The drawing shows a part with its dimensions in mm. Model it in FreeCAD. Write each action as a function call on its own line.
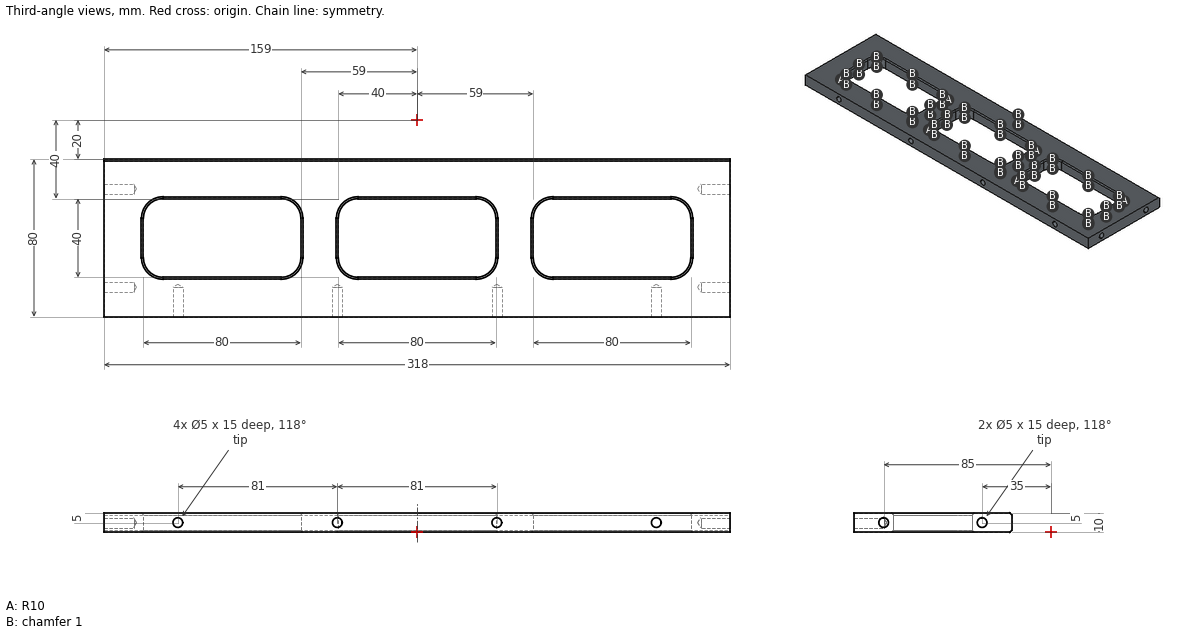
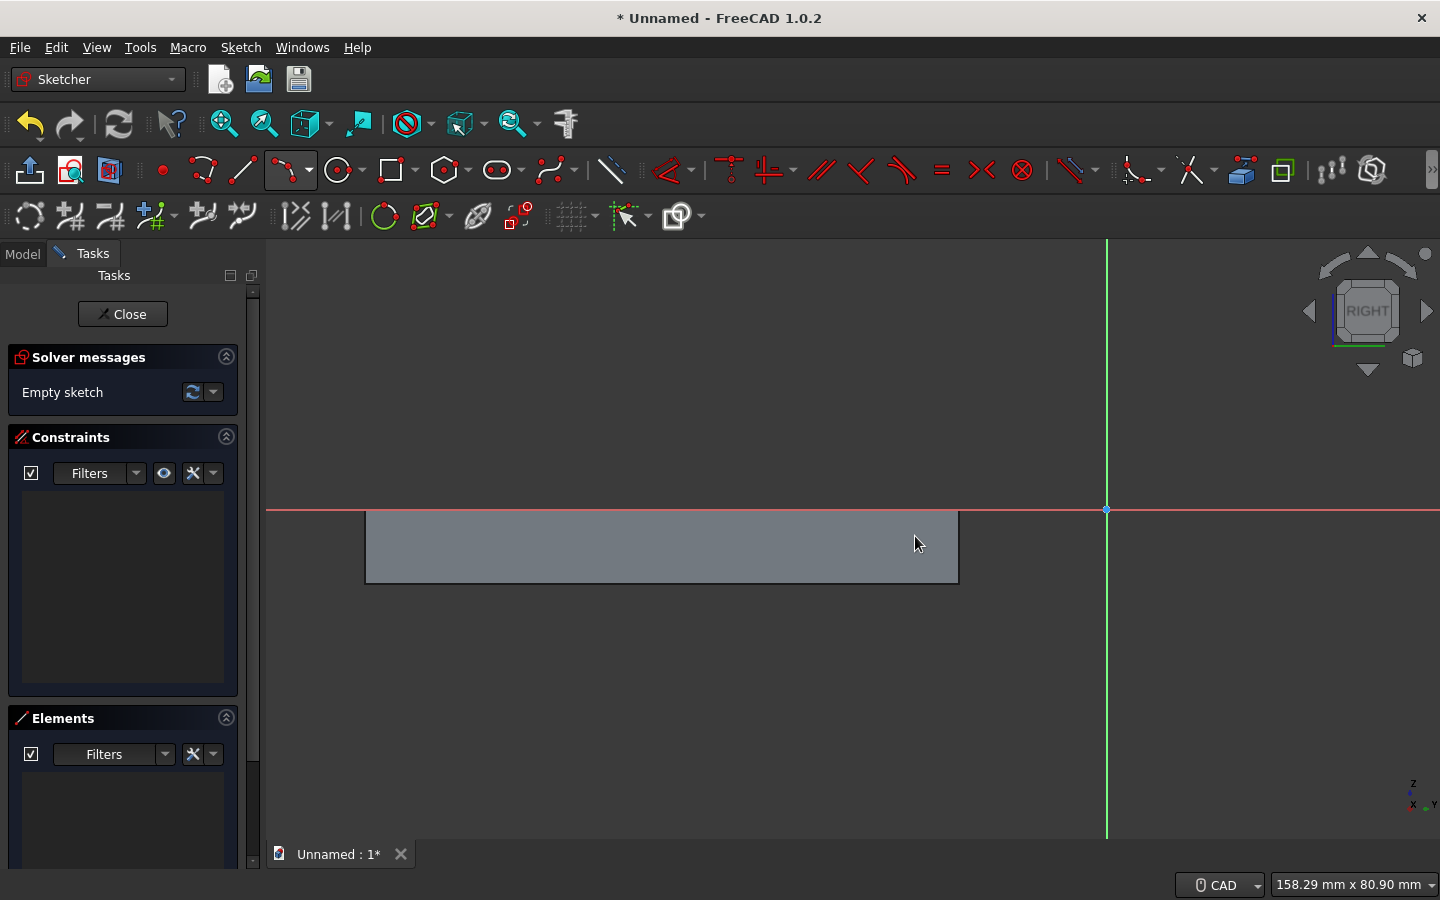
click(338, 170)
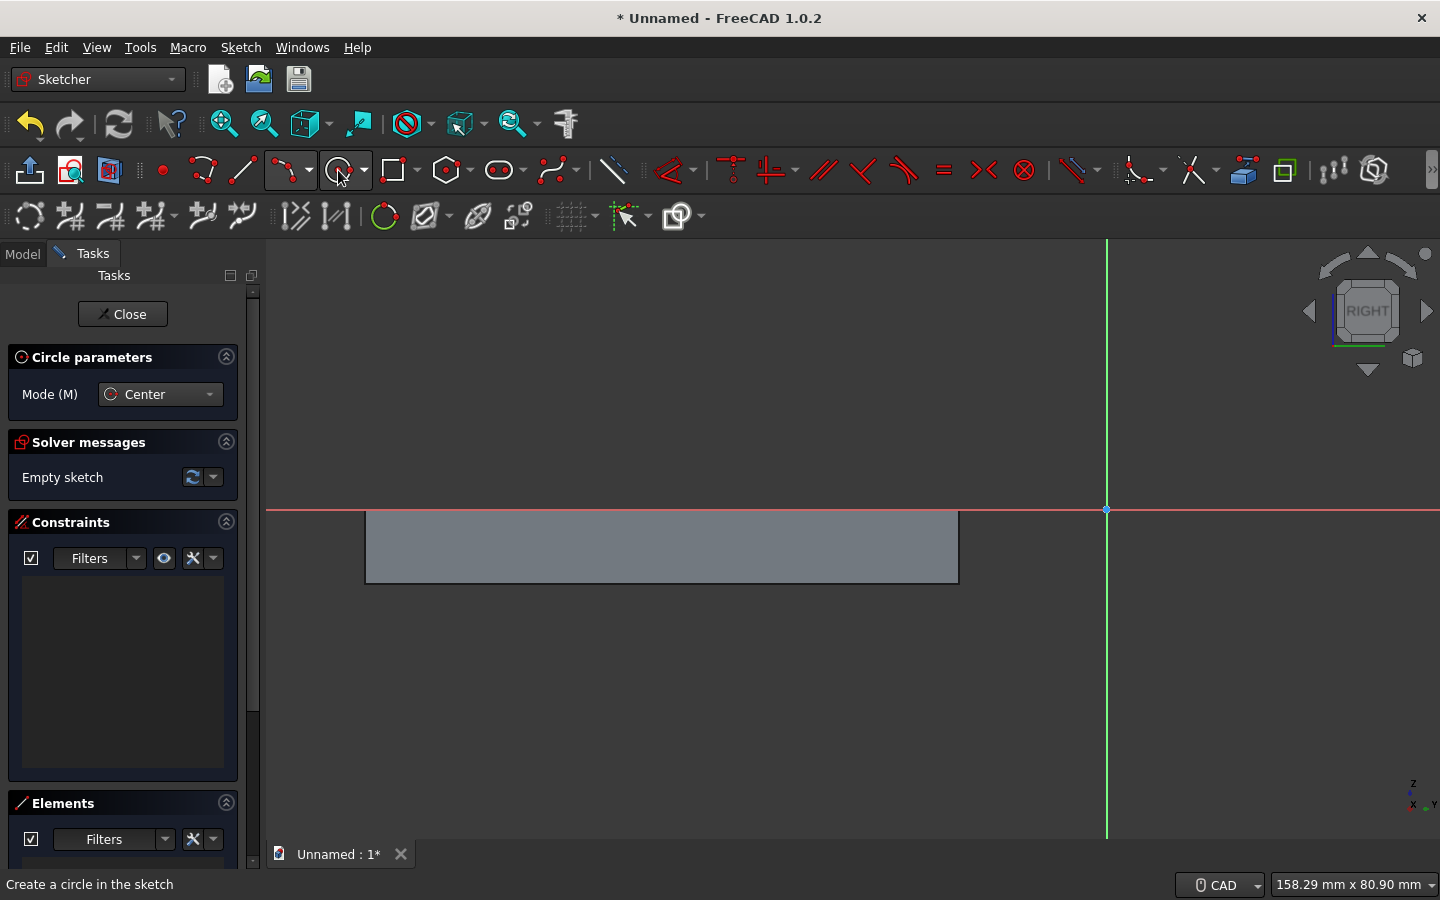
scroll(847, 547, up, 2)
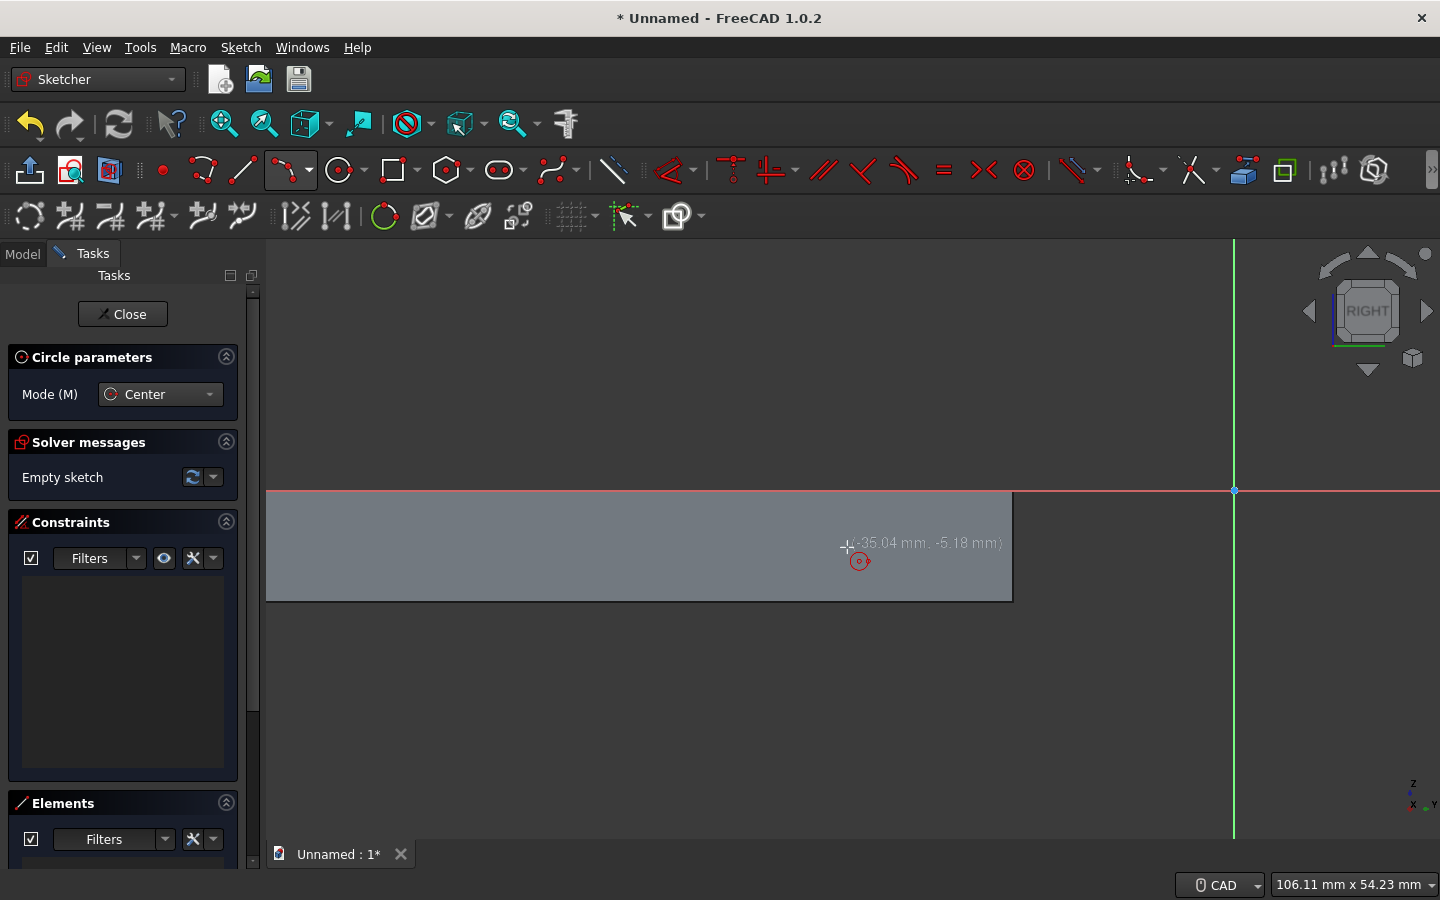
click(847, 546)
click(867, 527)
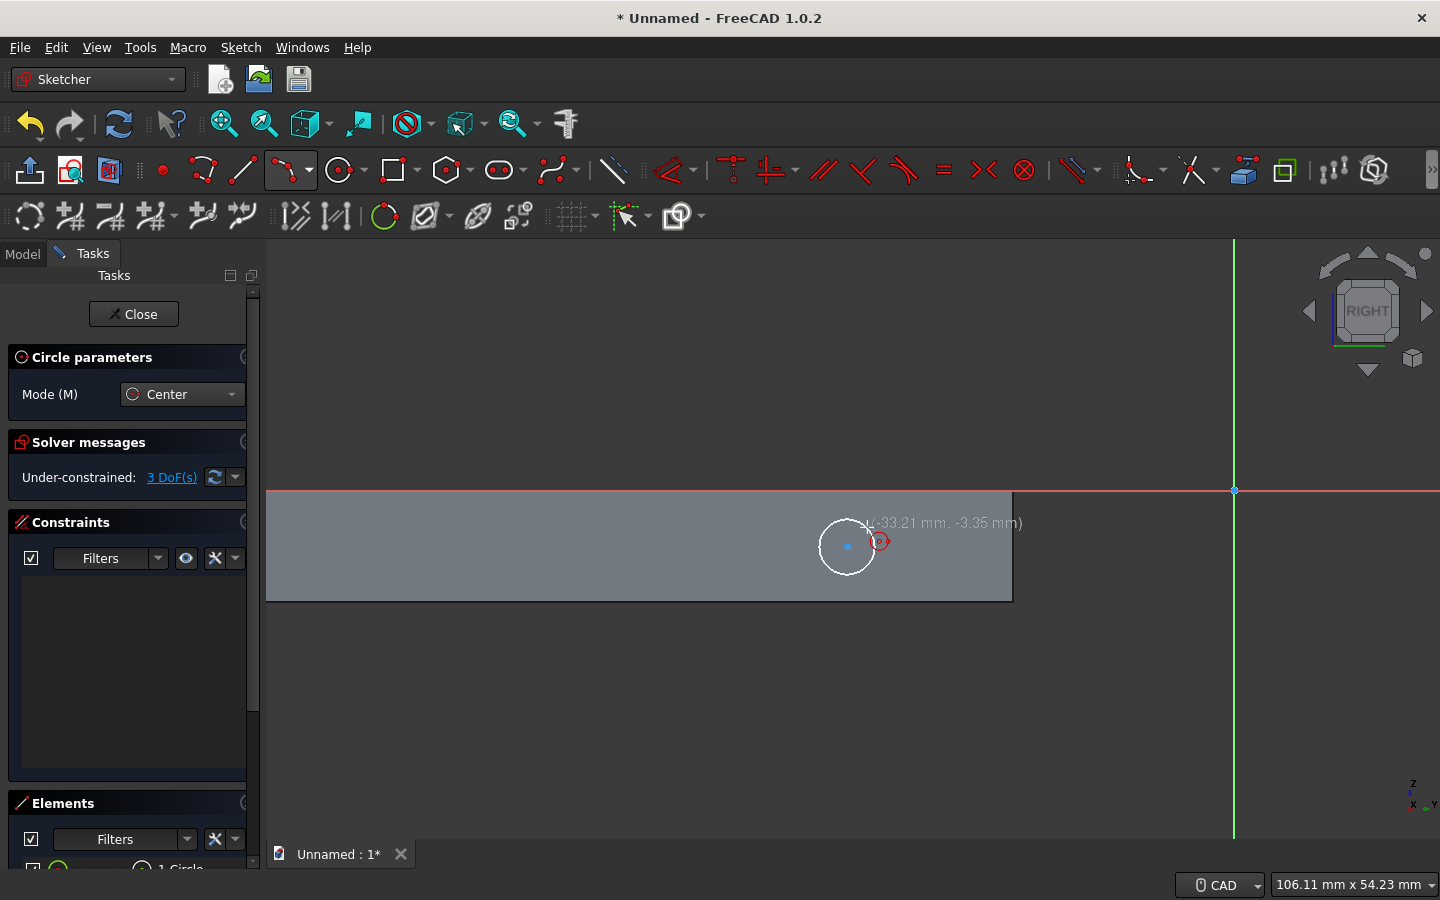
scroll(854, 552, down, 2)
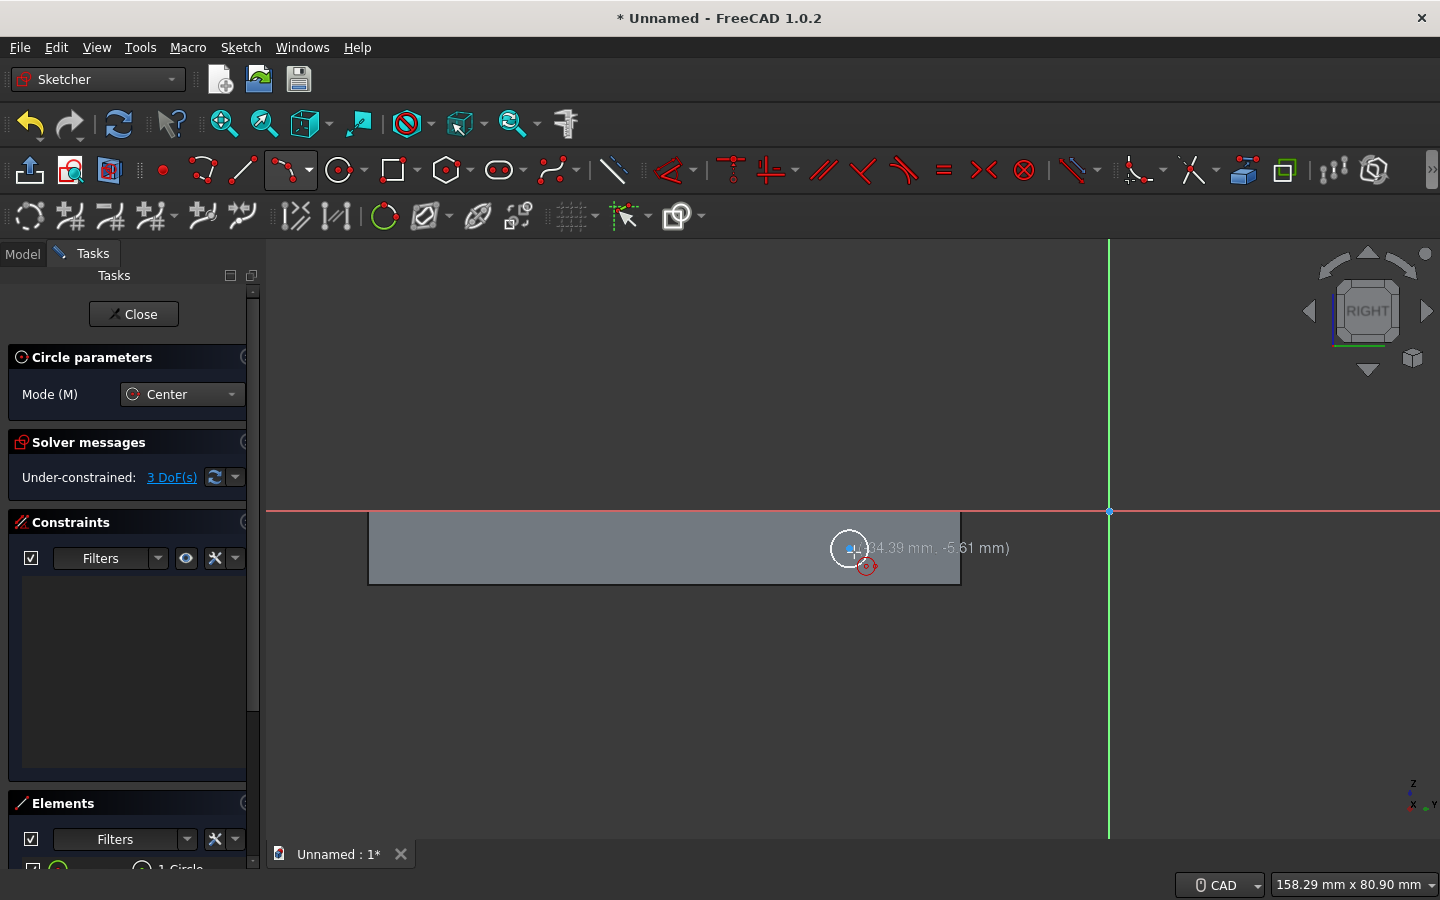
scroll(479, 548, up, 2)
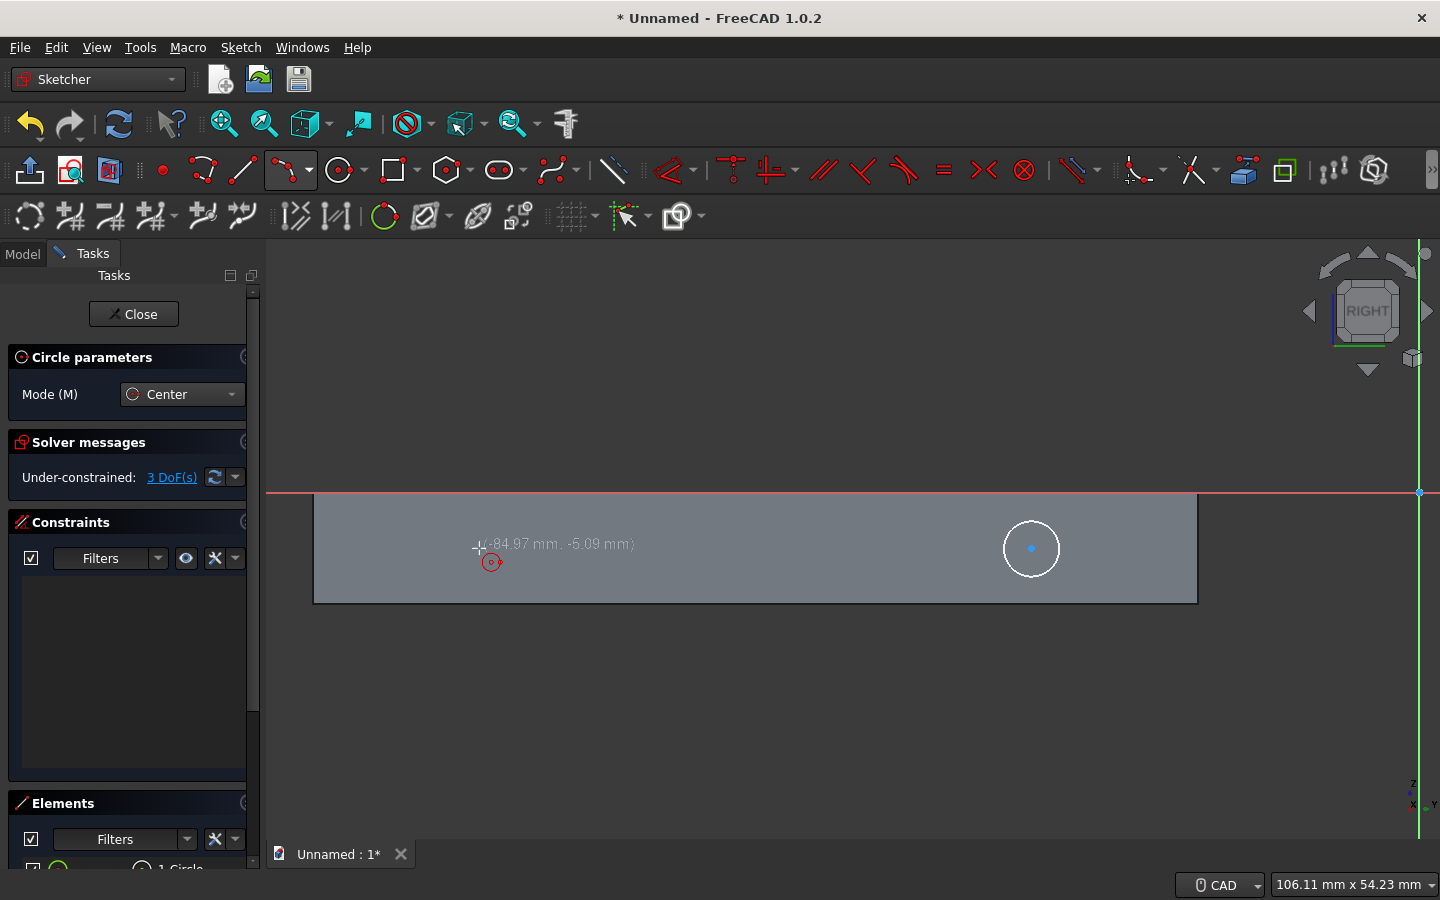
click(479, 548)
click(498, 529)
key(Escape)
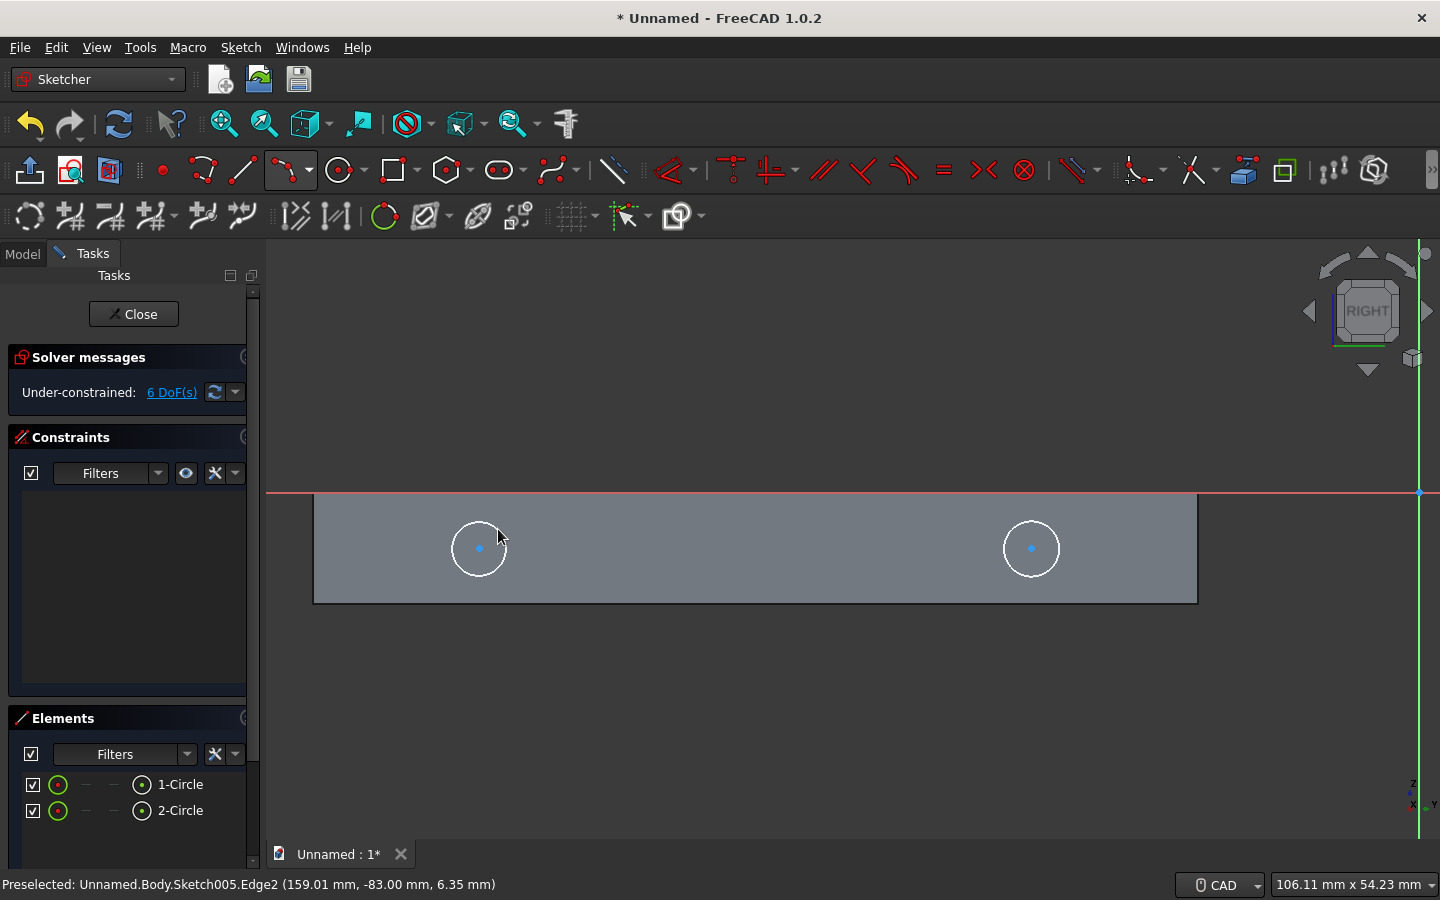
click(1051, 529)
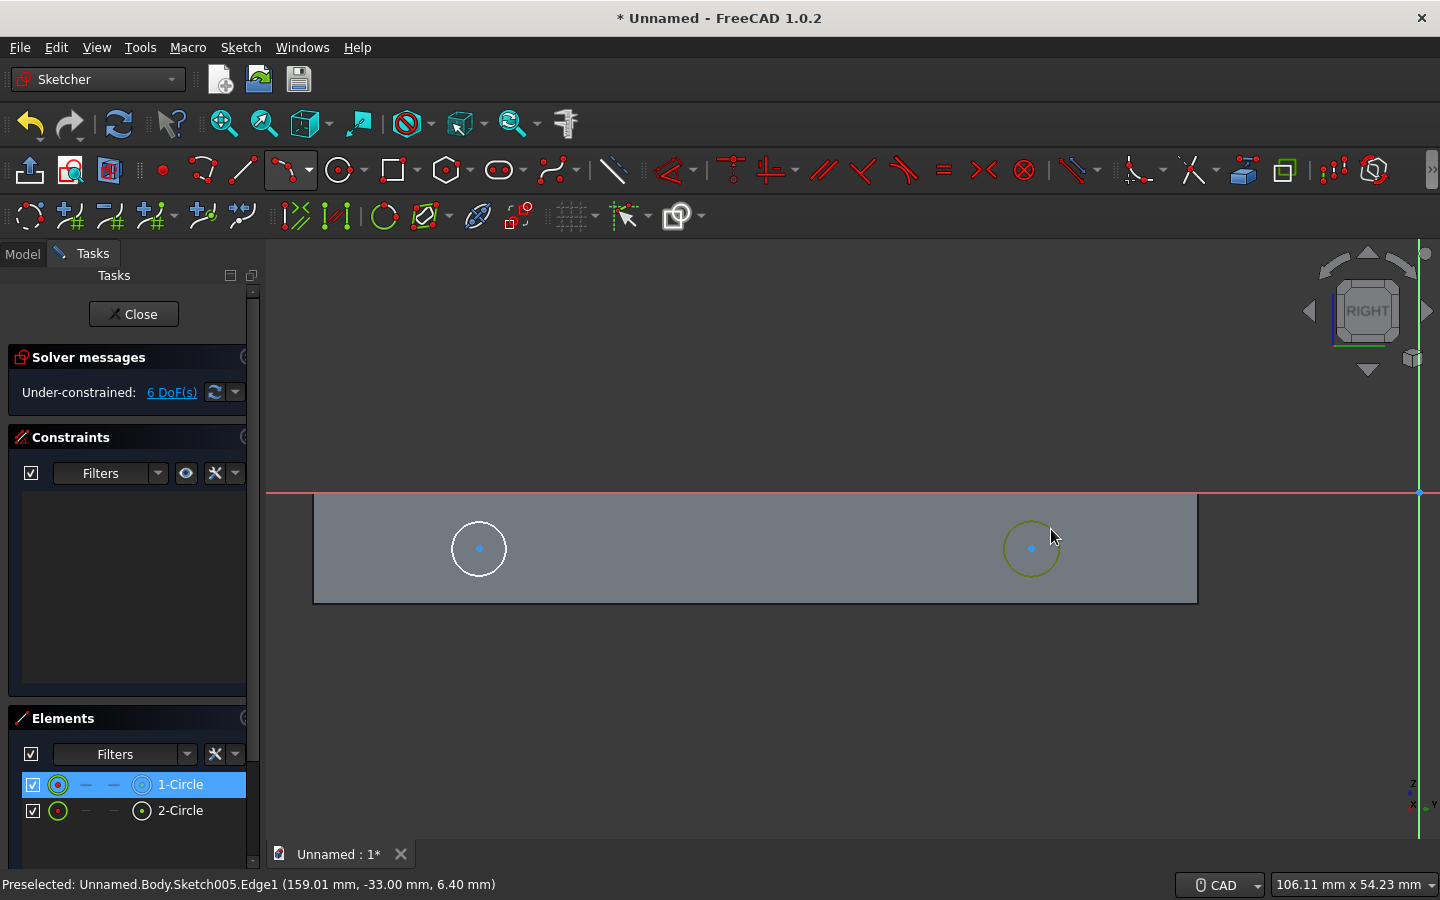
click(498, 530)